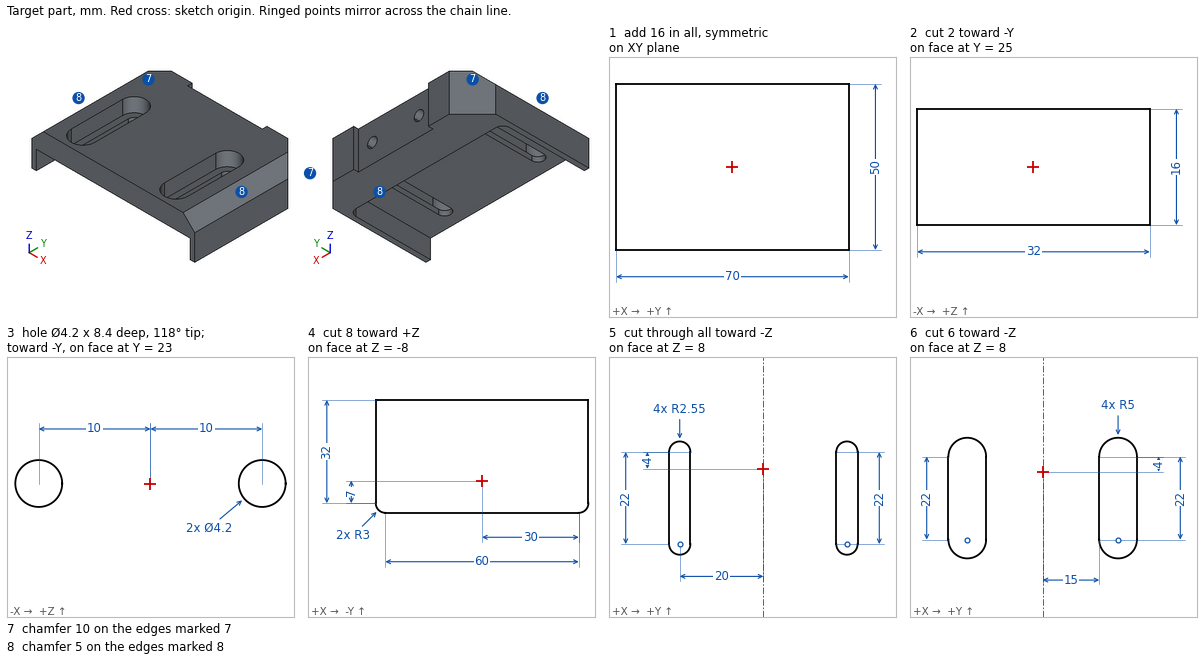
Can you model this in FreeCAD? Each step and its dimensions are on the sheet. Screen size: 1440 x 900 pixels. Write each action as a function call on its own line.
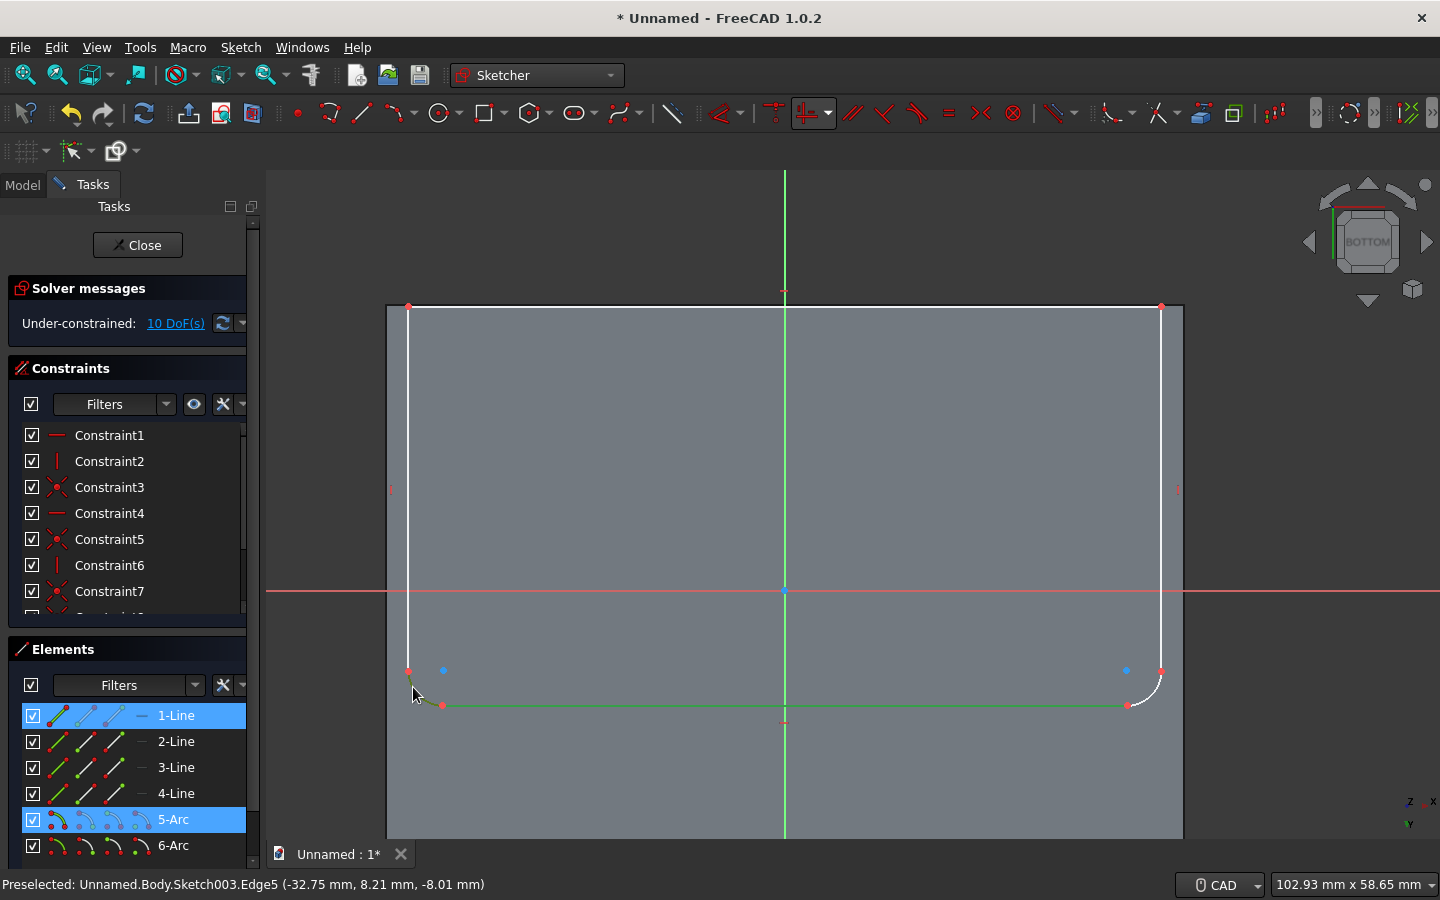
click(918, 114)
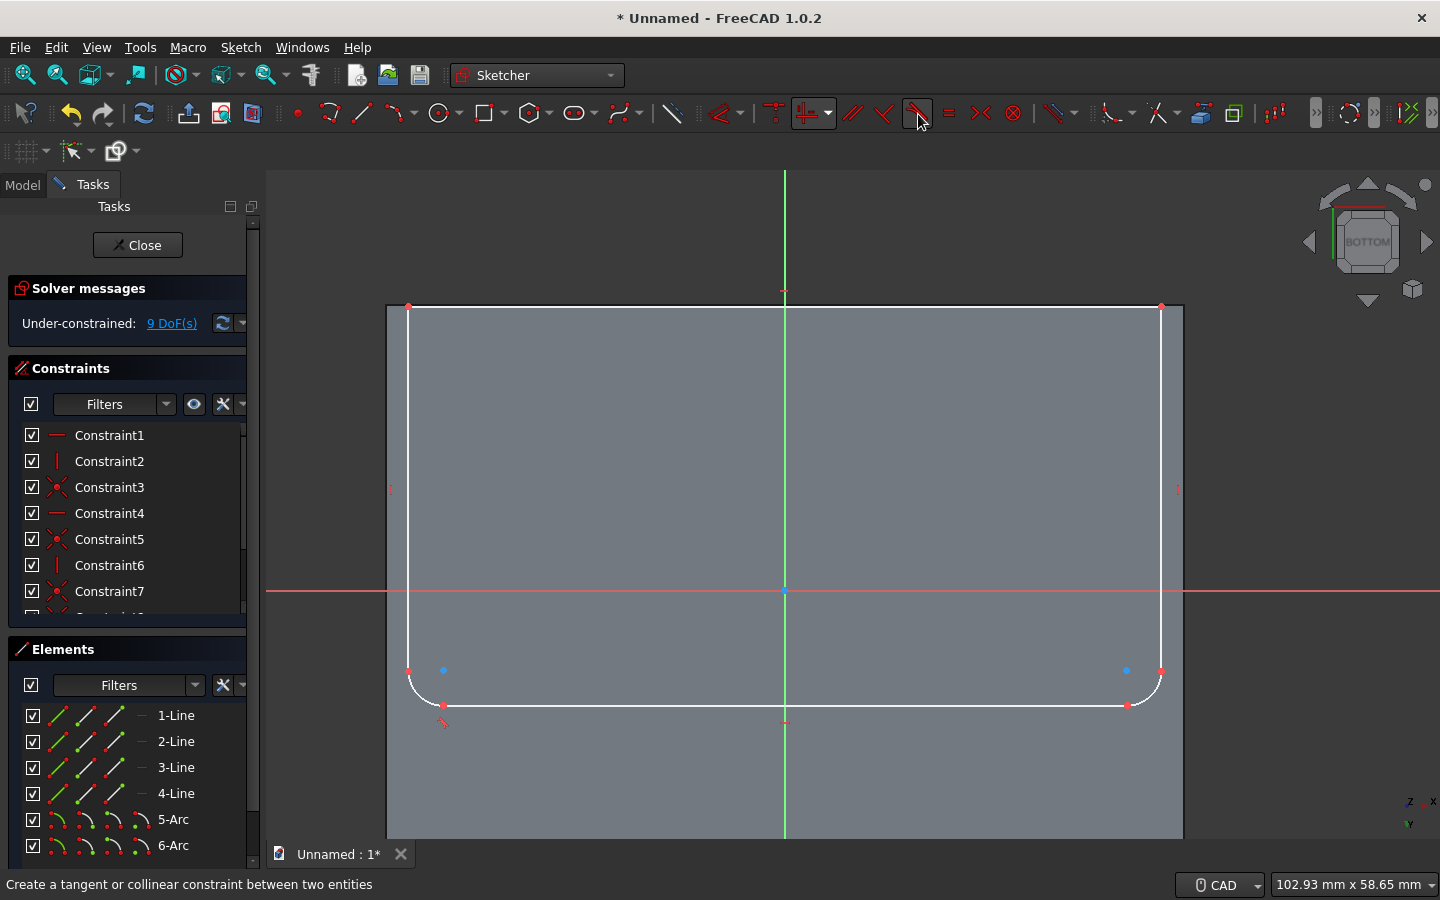
click(922, 706)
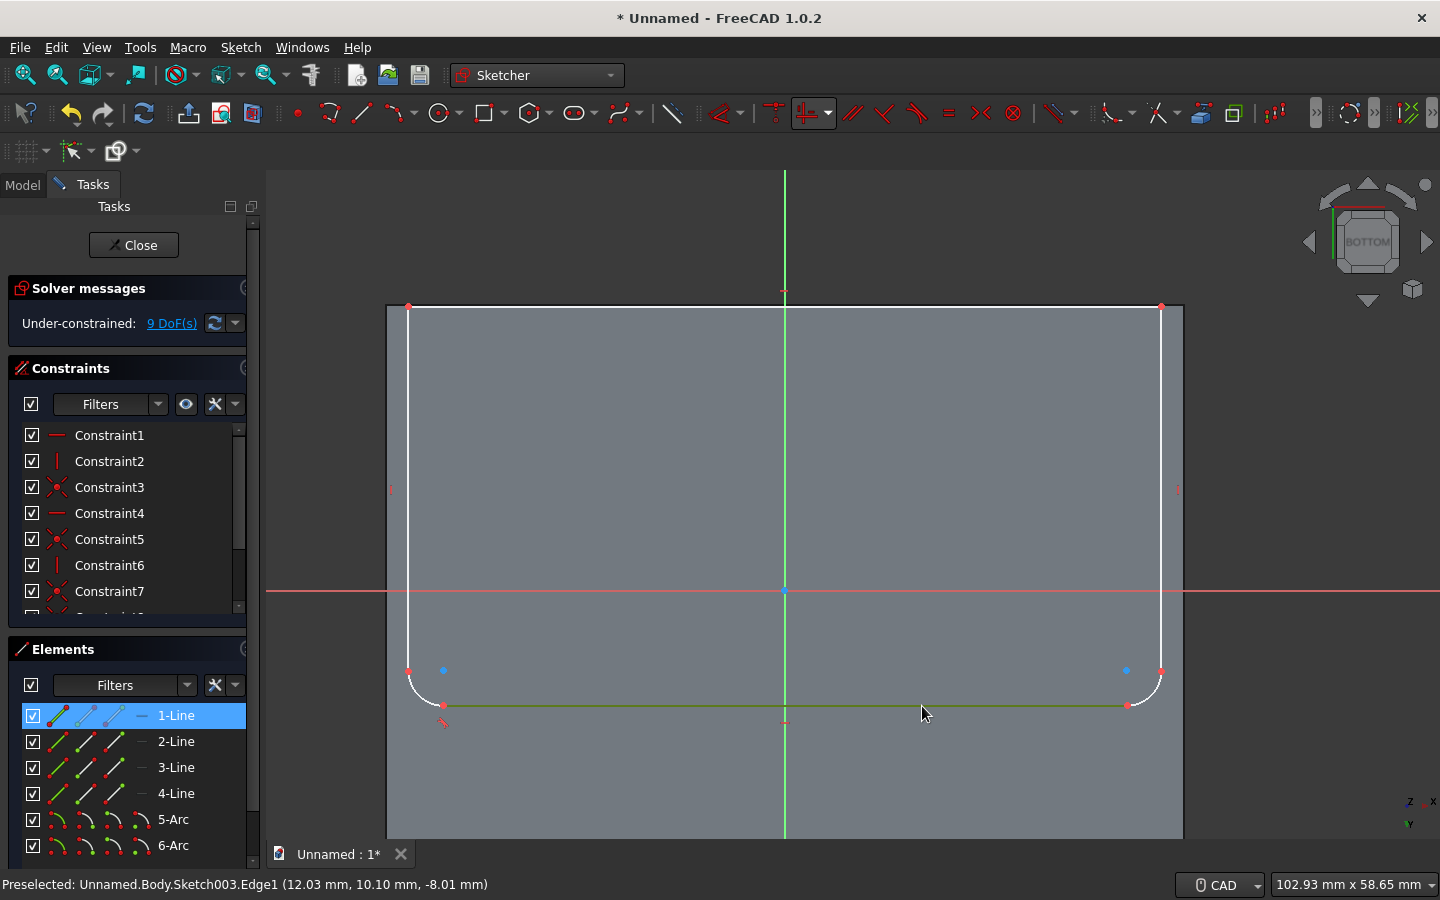
click(1143, 702)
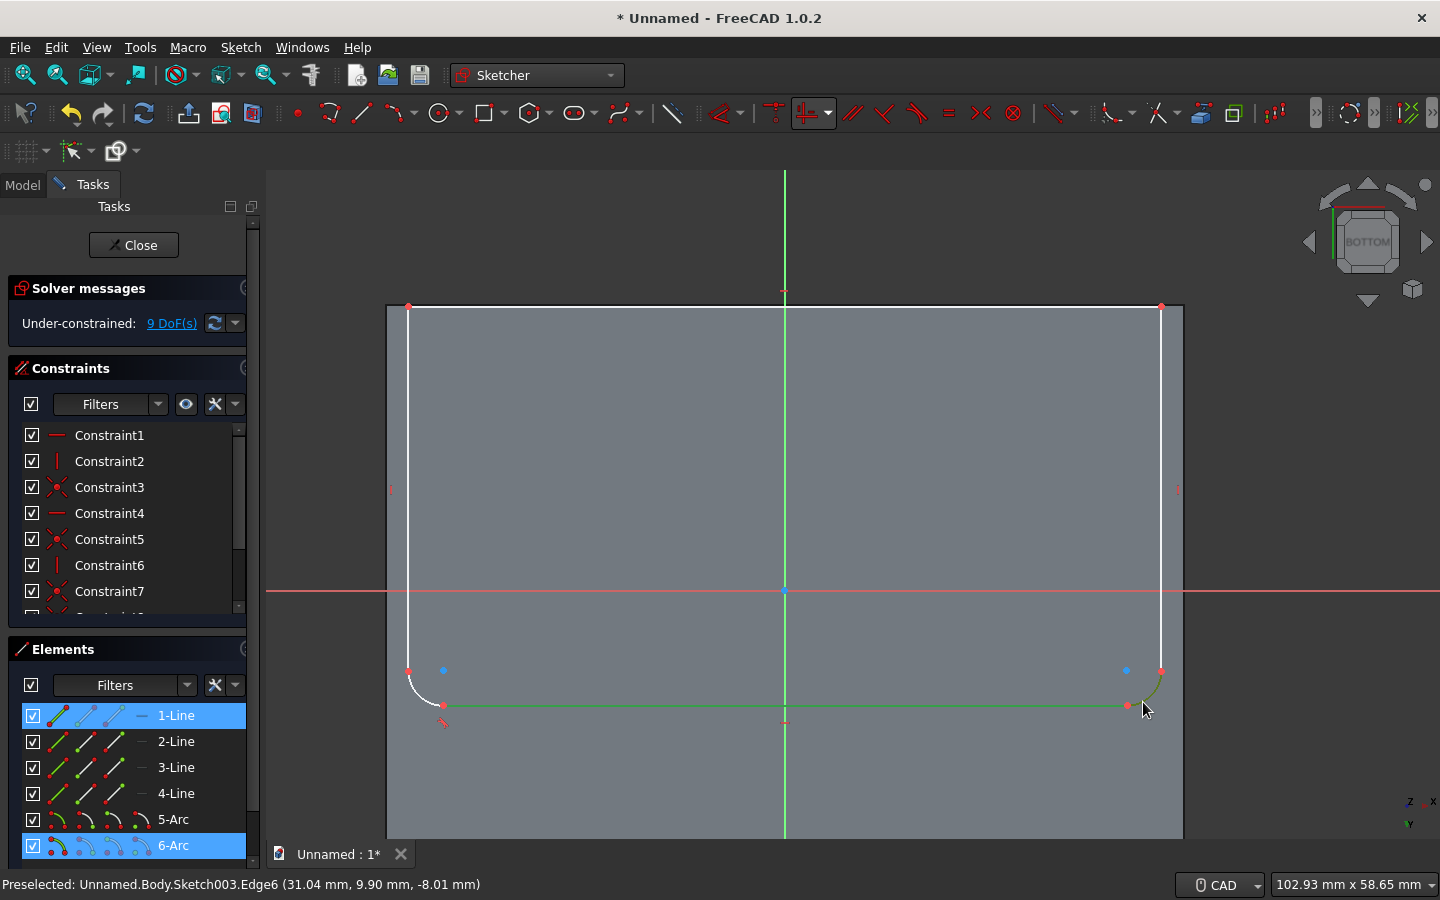
key(t)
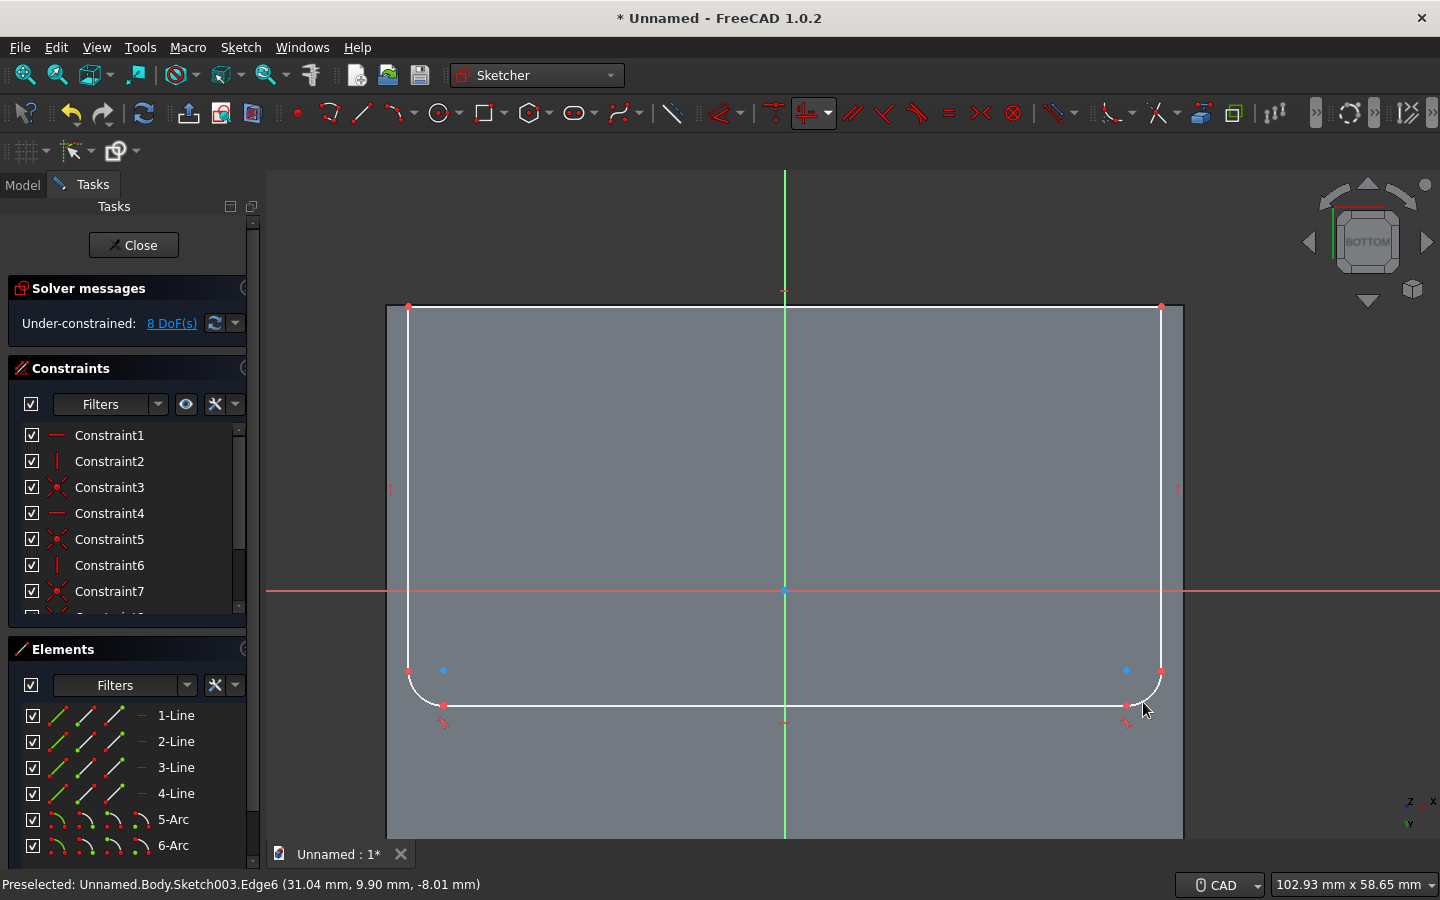
click(408, 562)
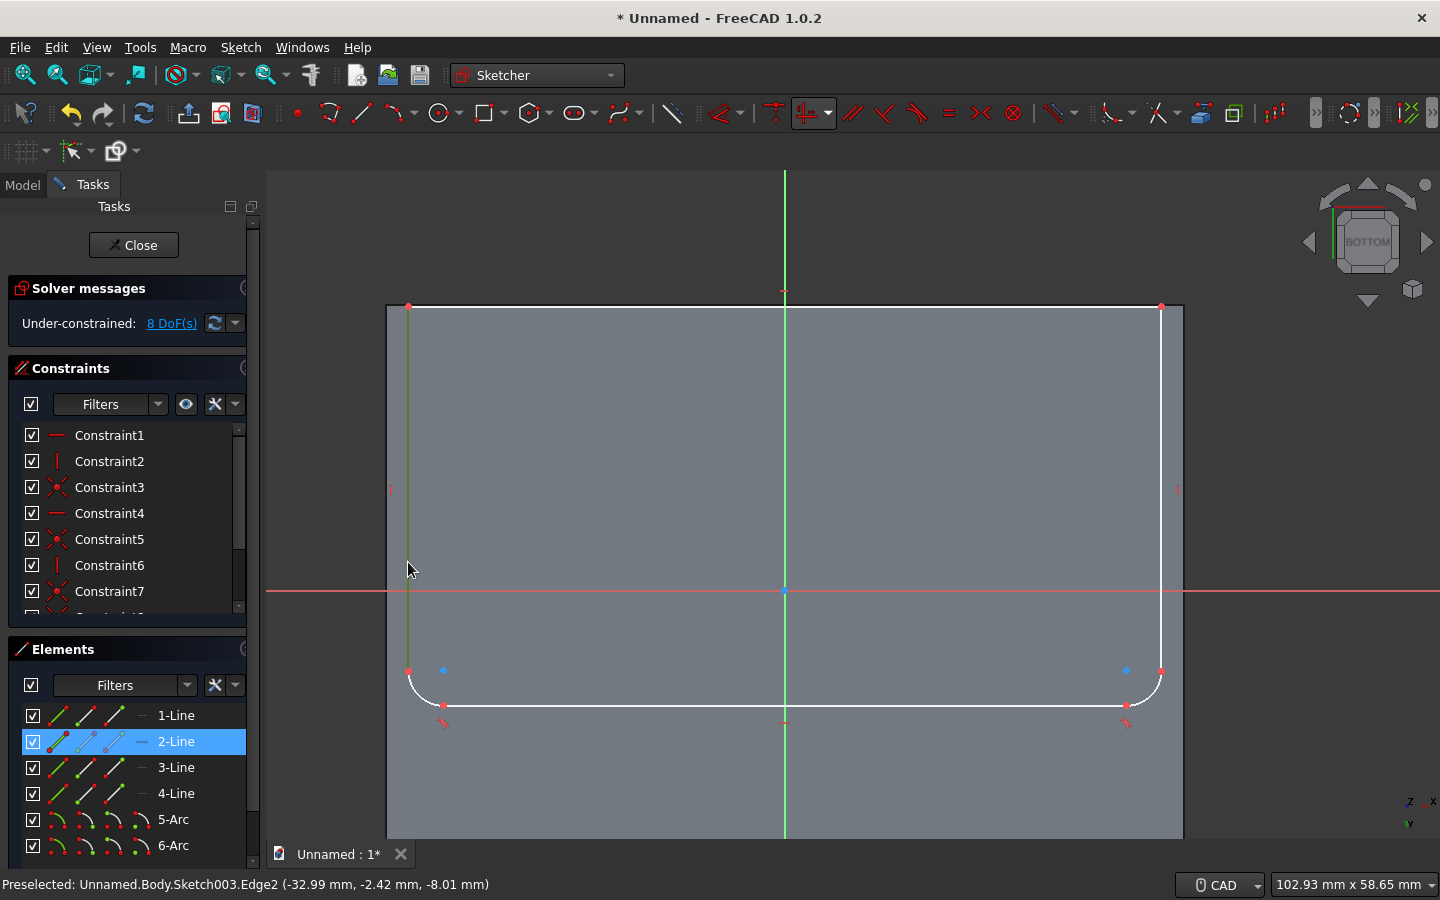
click(413, 687)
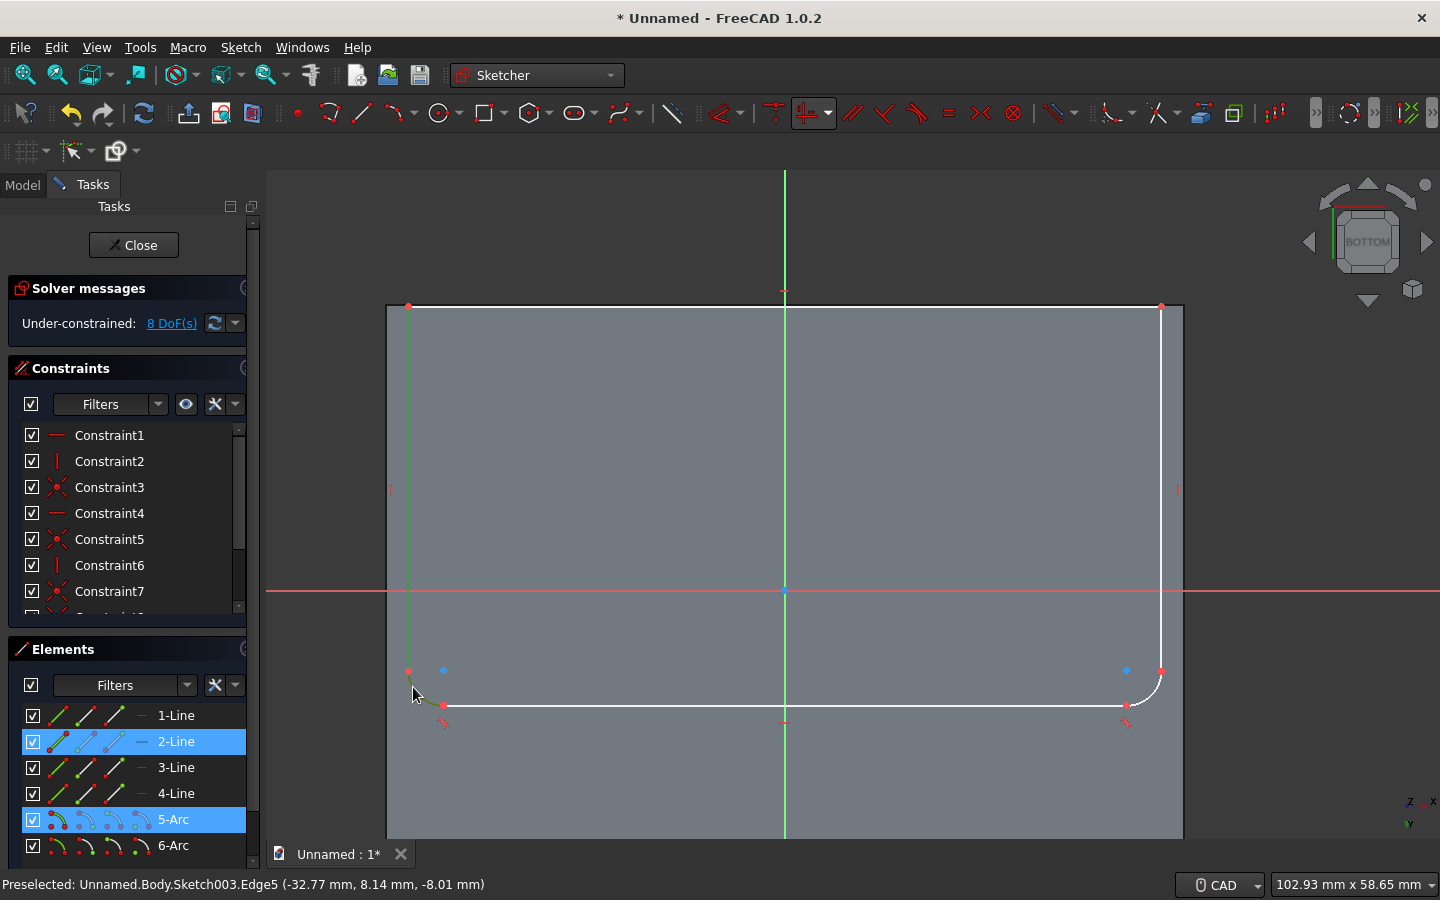
key(t)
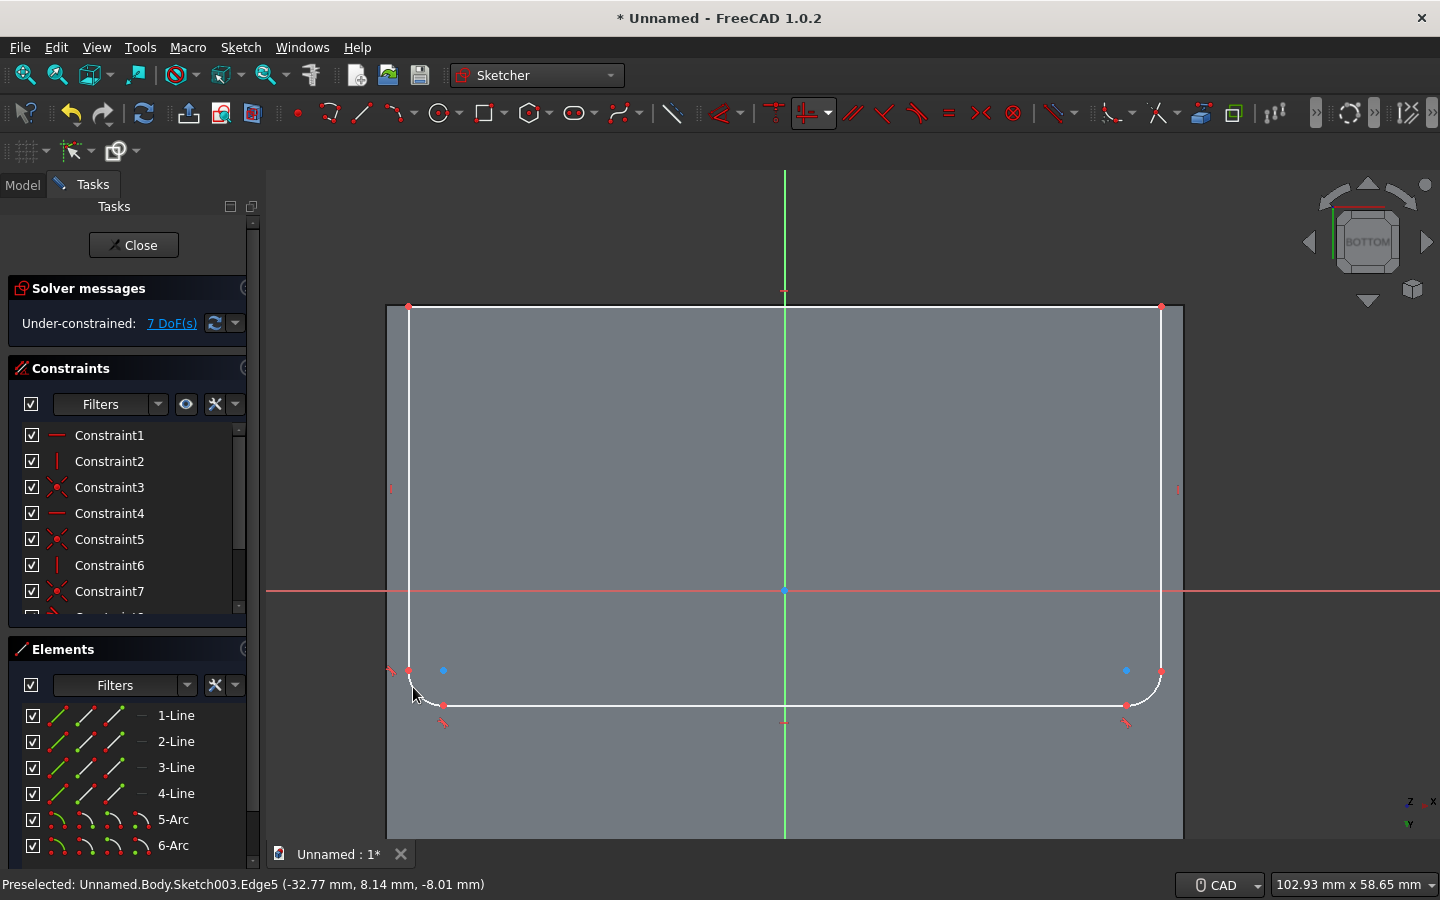
click(1161, 416)